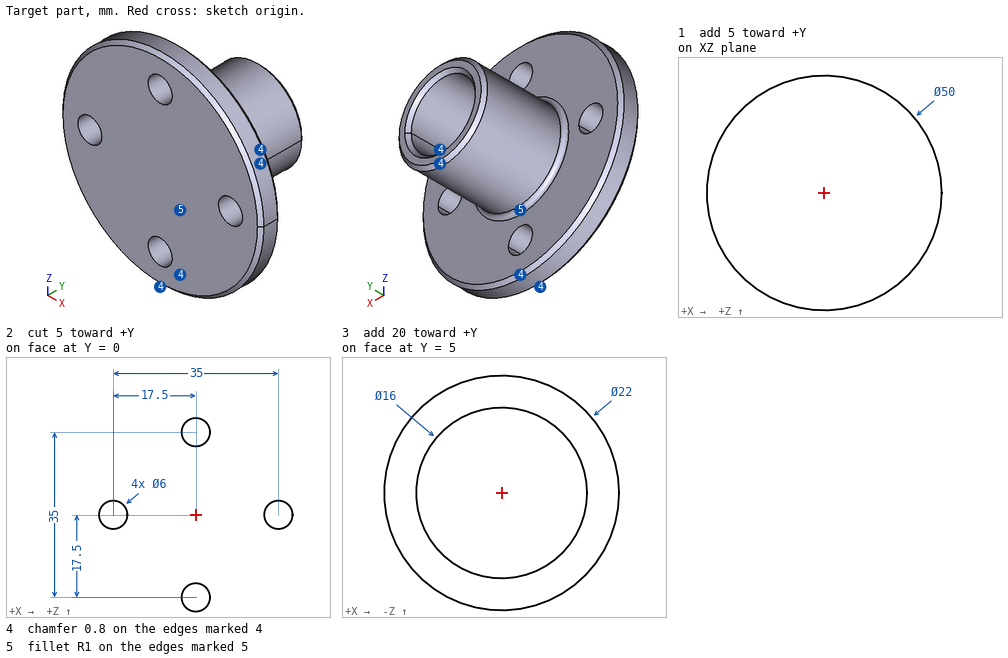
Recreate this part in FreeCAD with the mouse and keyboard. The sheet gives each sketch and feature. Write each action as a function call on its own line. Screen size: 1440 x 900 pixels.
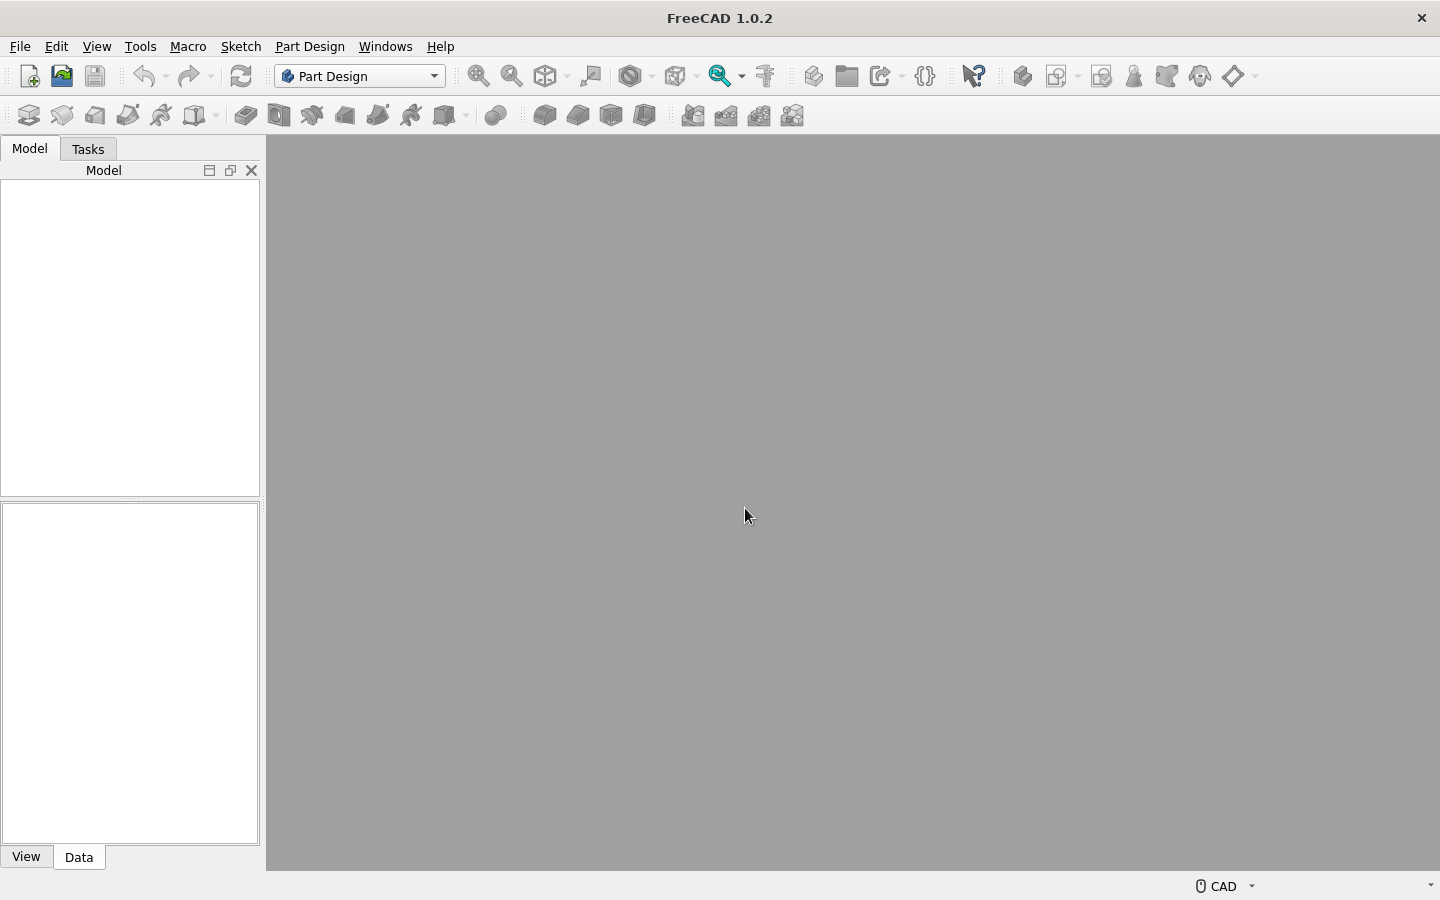
click(29, 76)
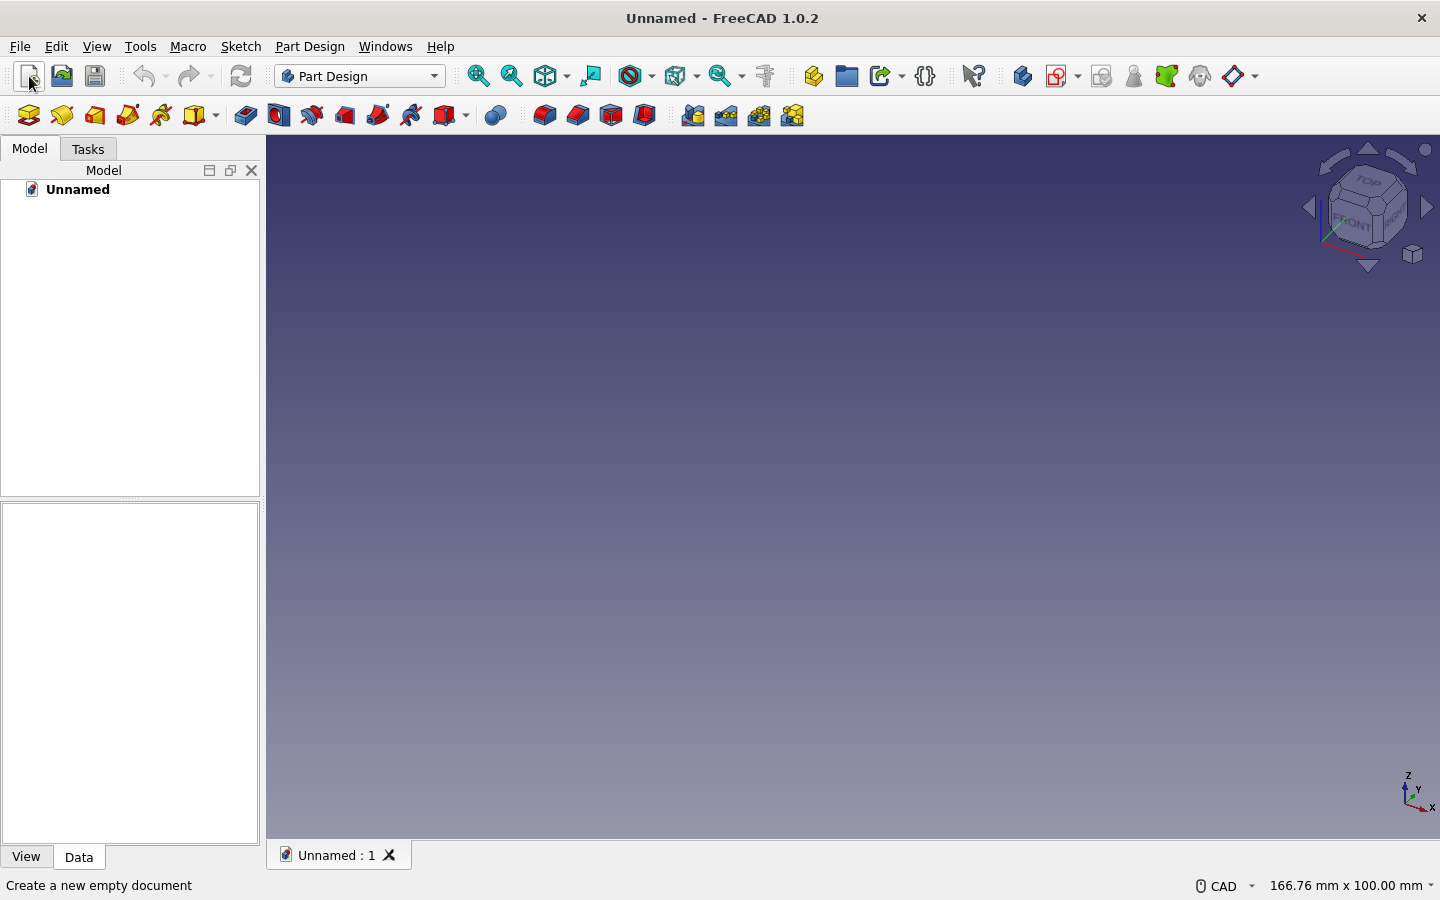
click(1056, 76)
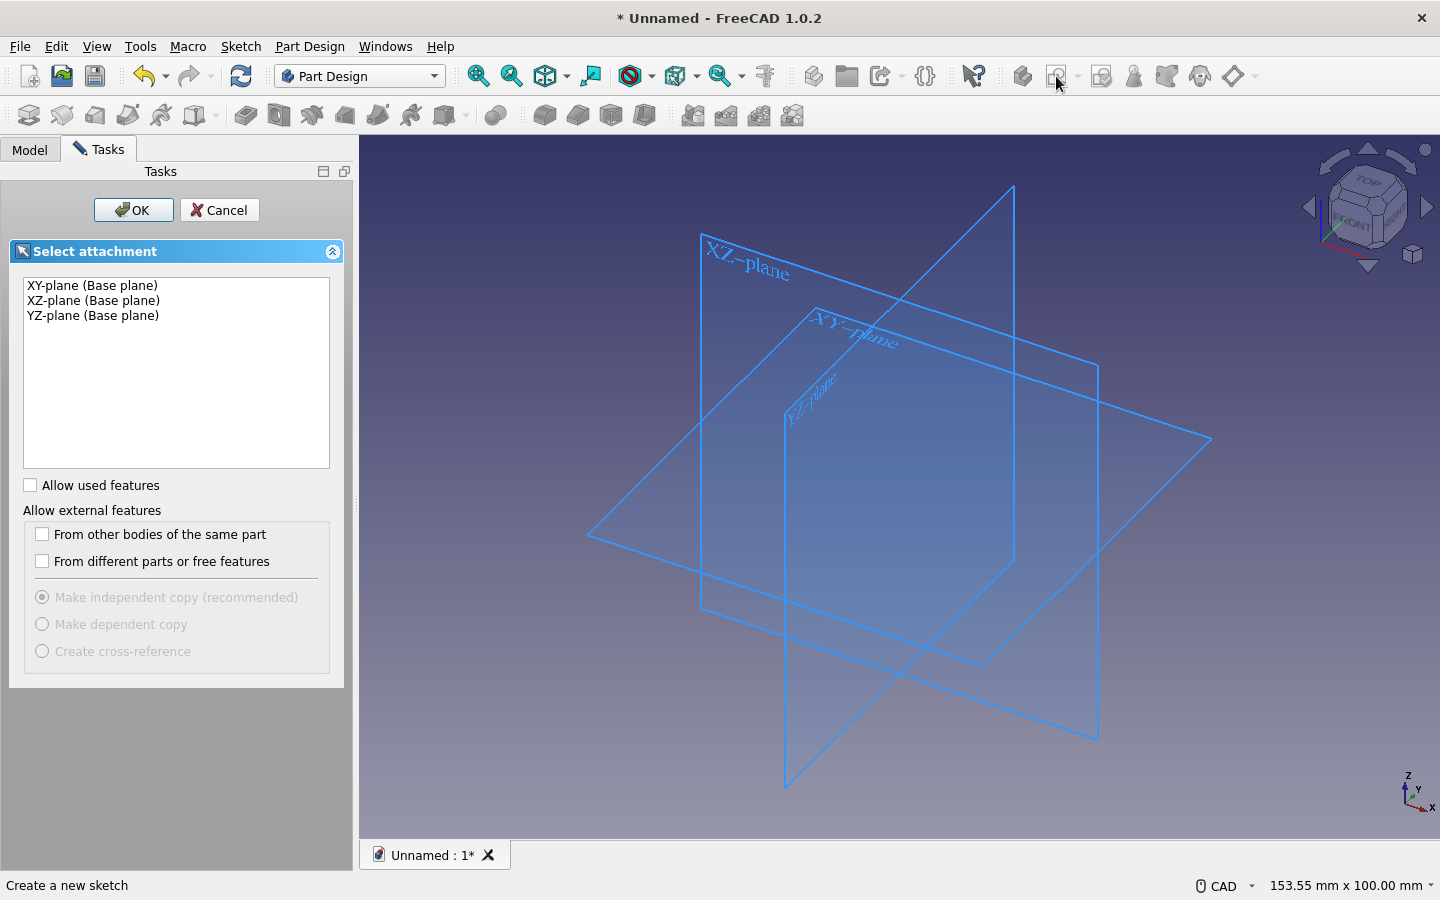
click(84, 300)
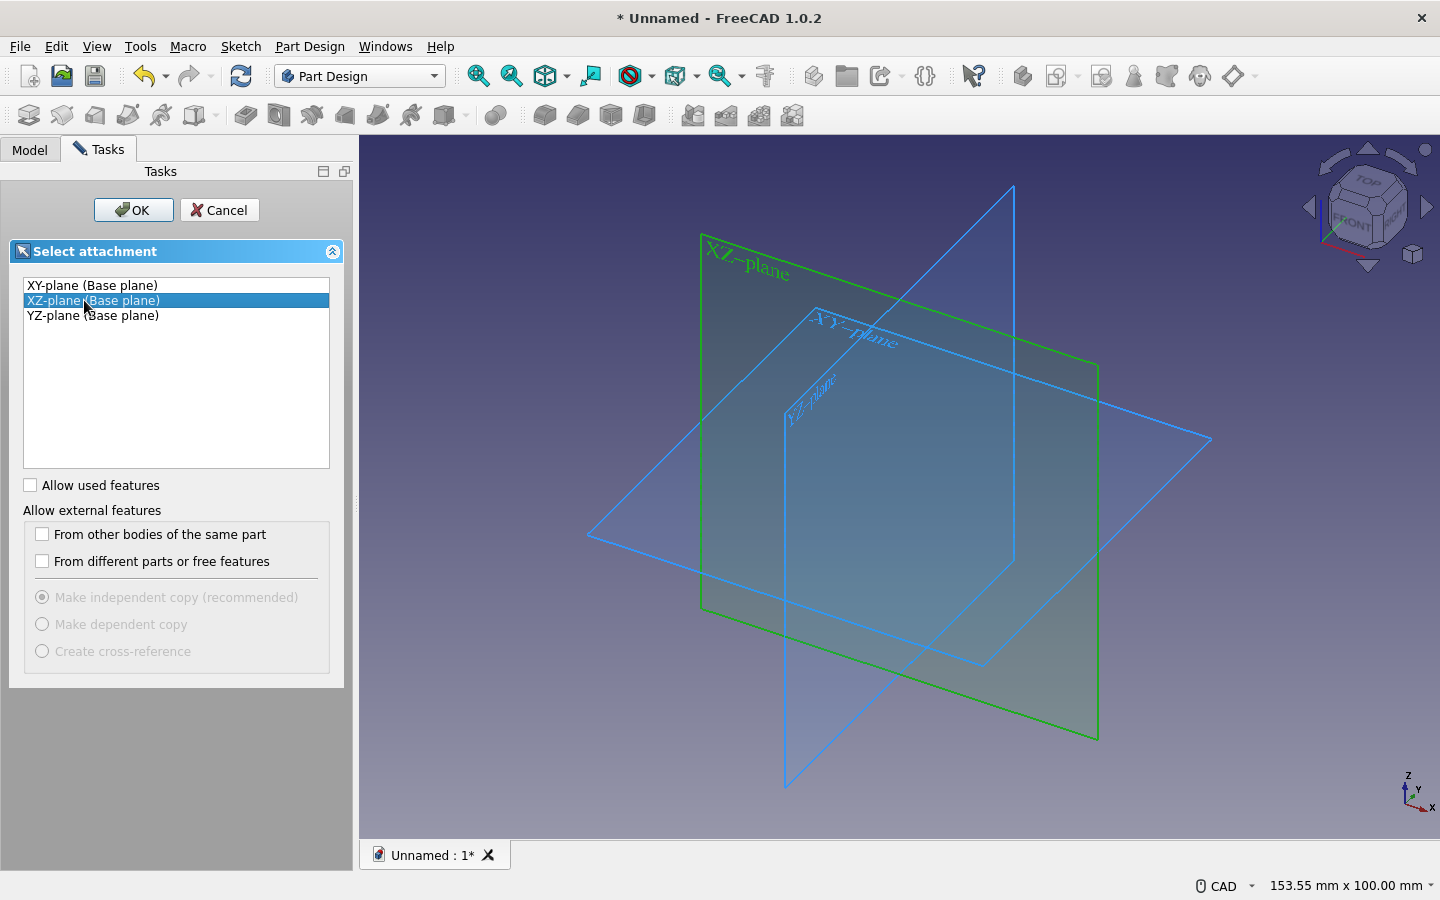
click(134, 210)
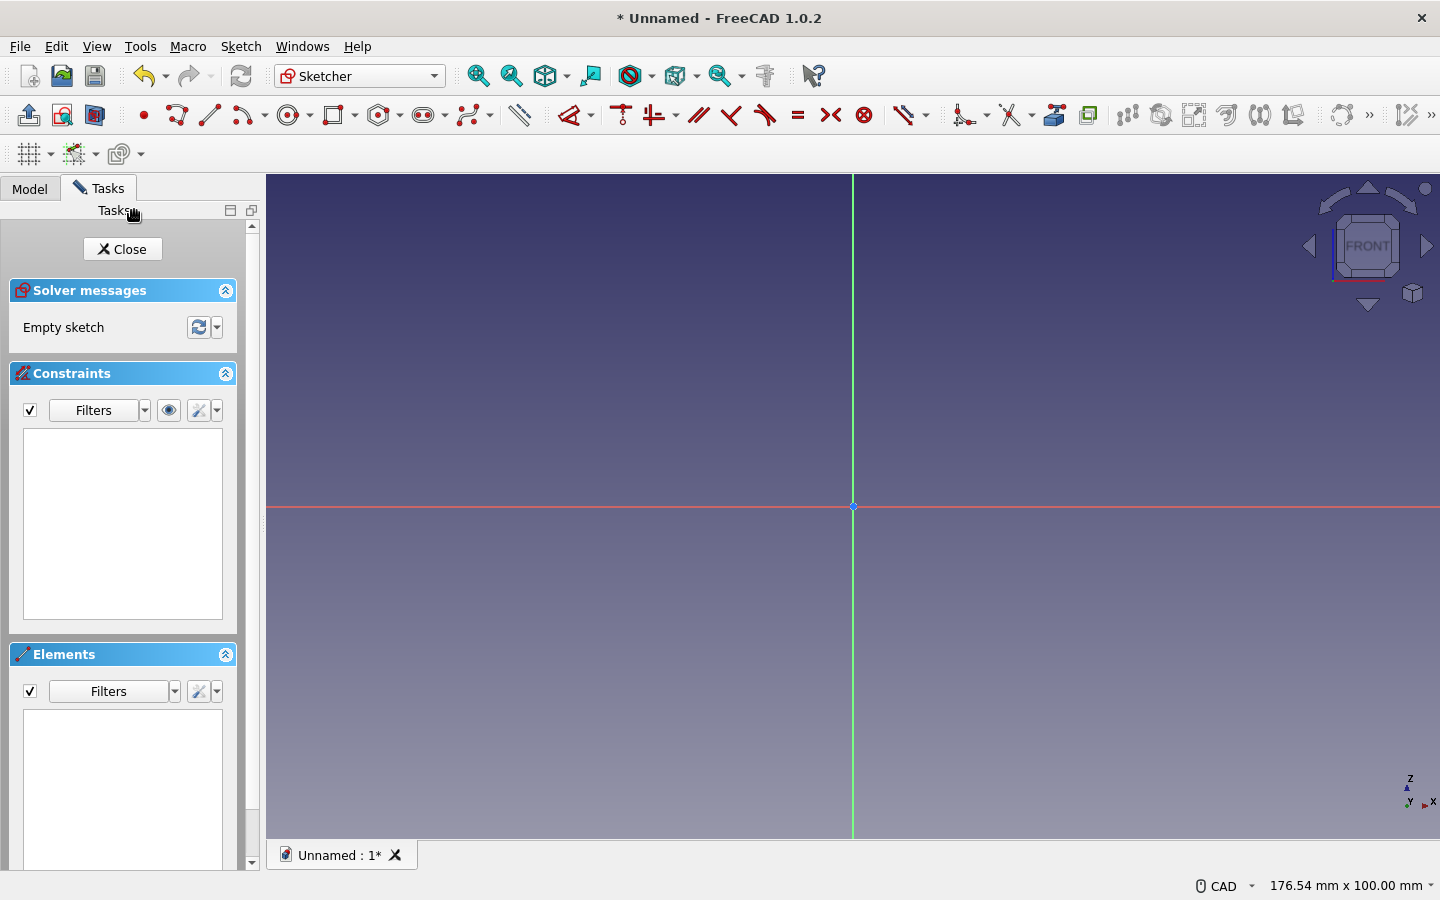
click(288, 116)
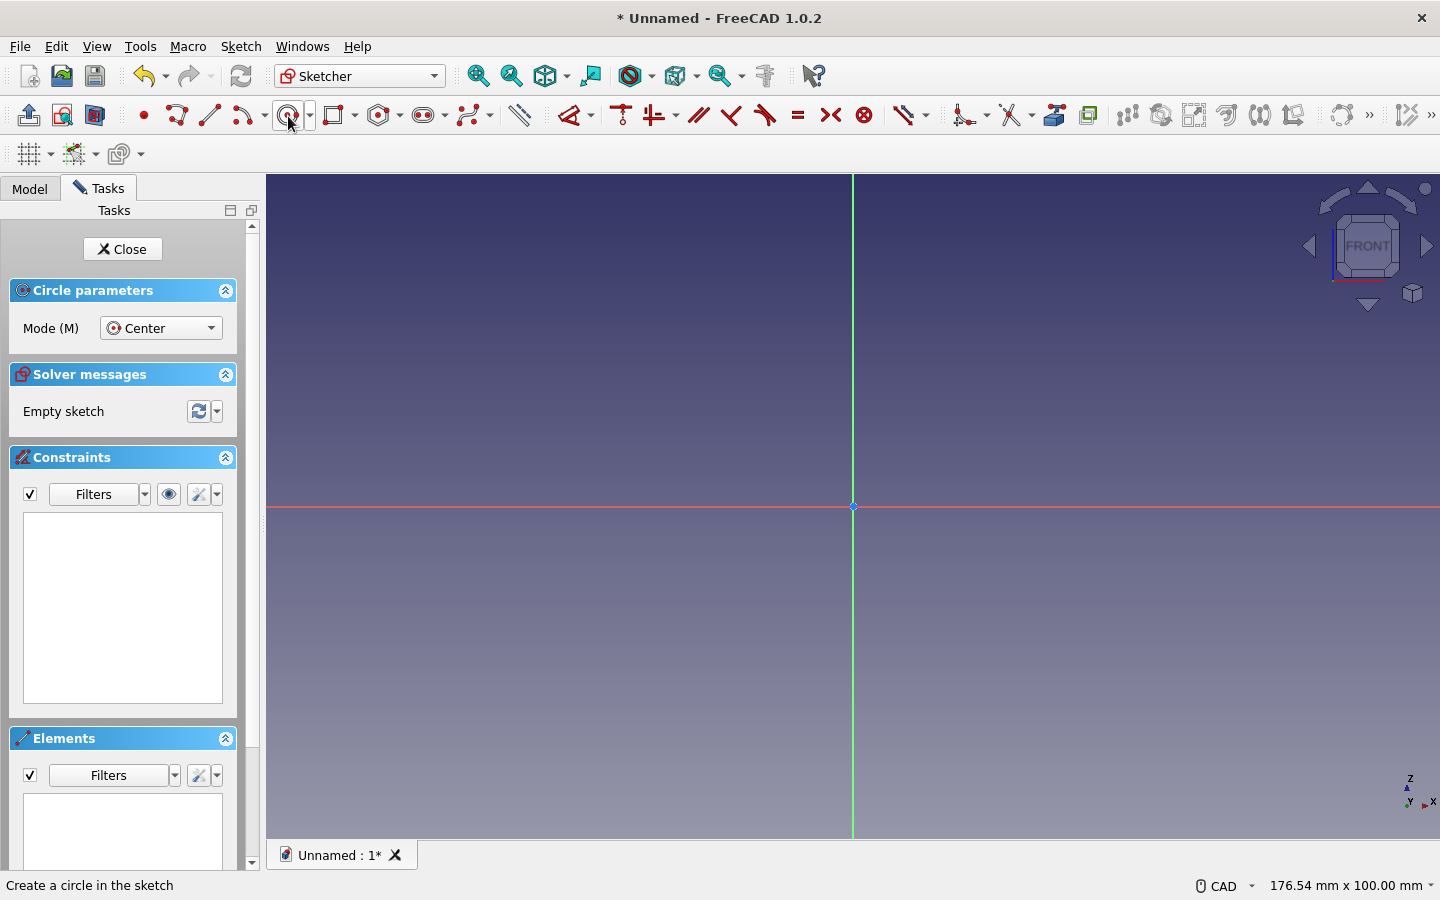
click(853, 506)
click(971, 389)
key(Escape)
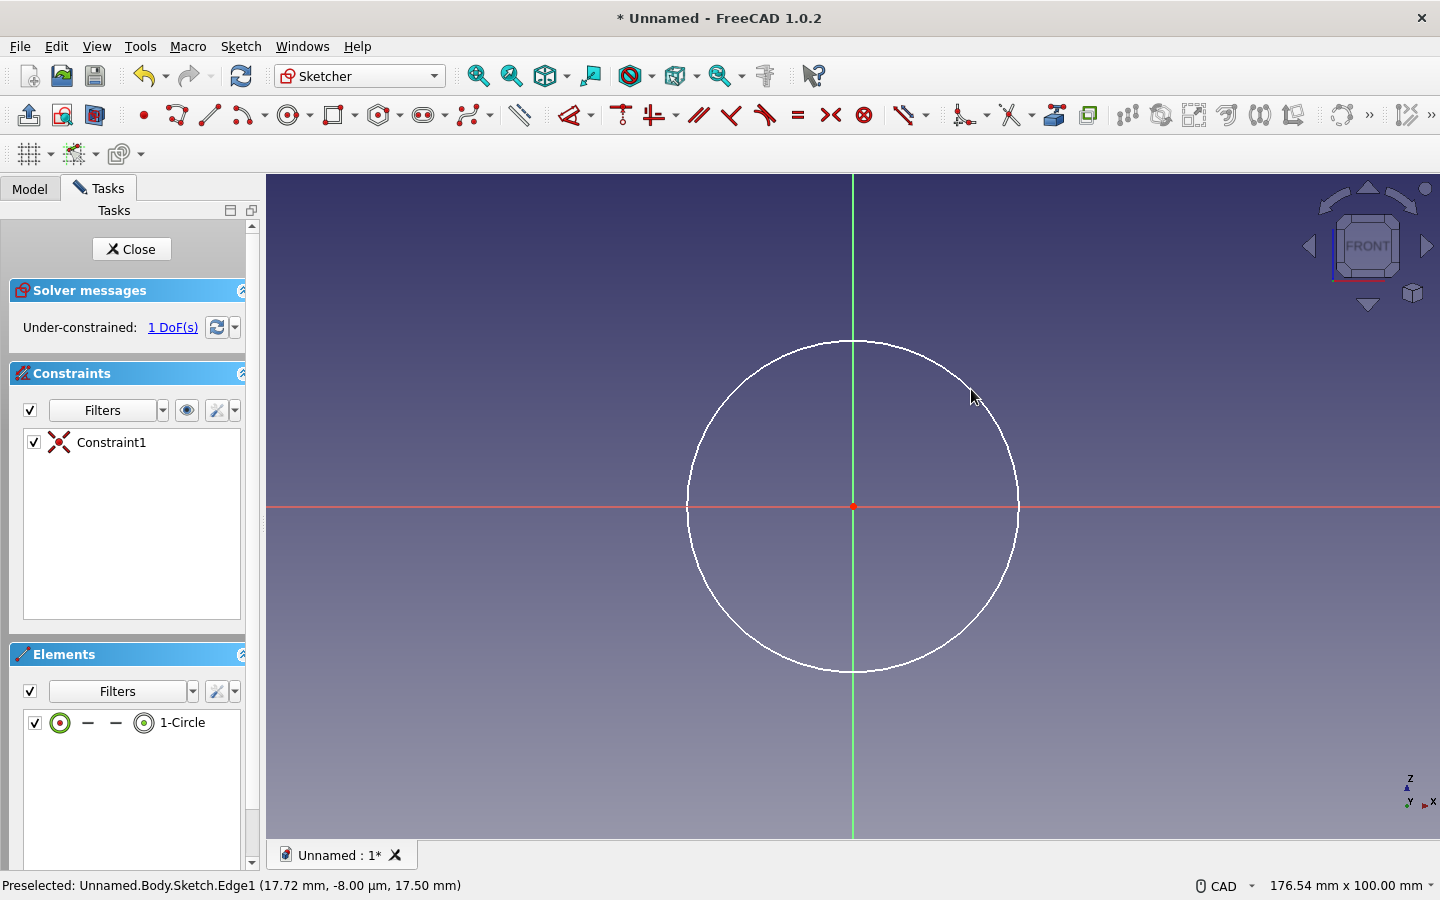
click(568, 116)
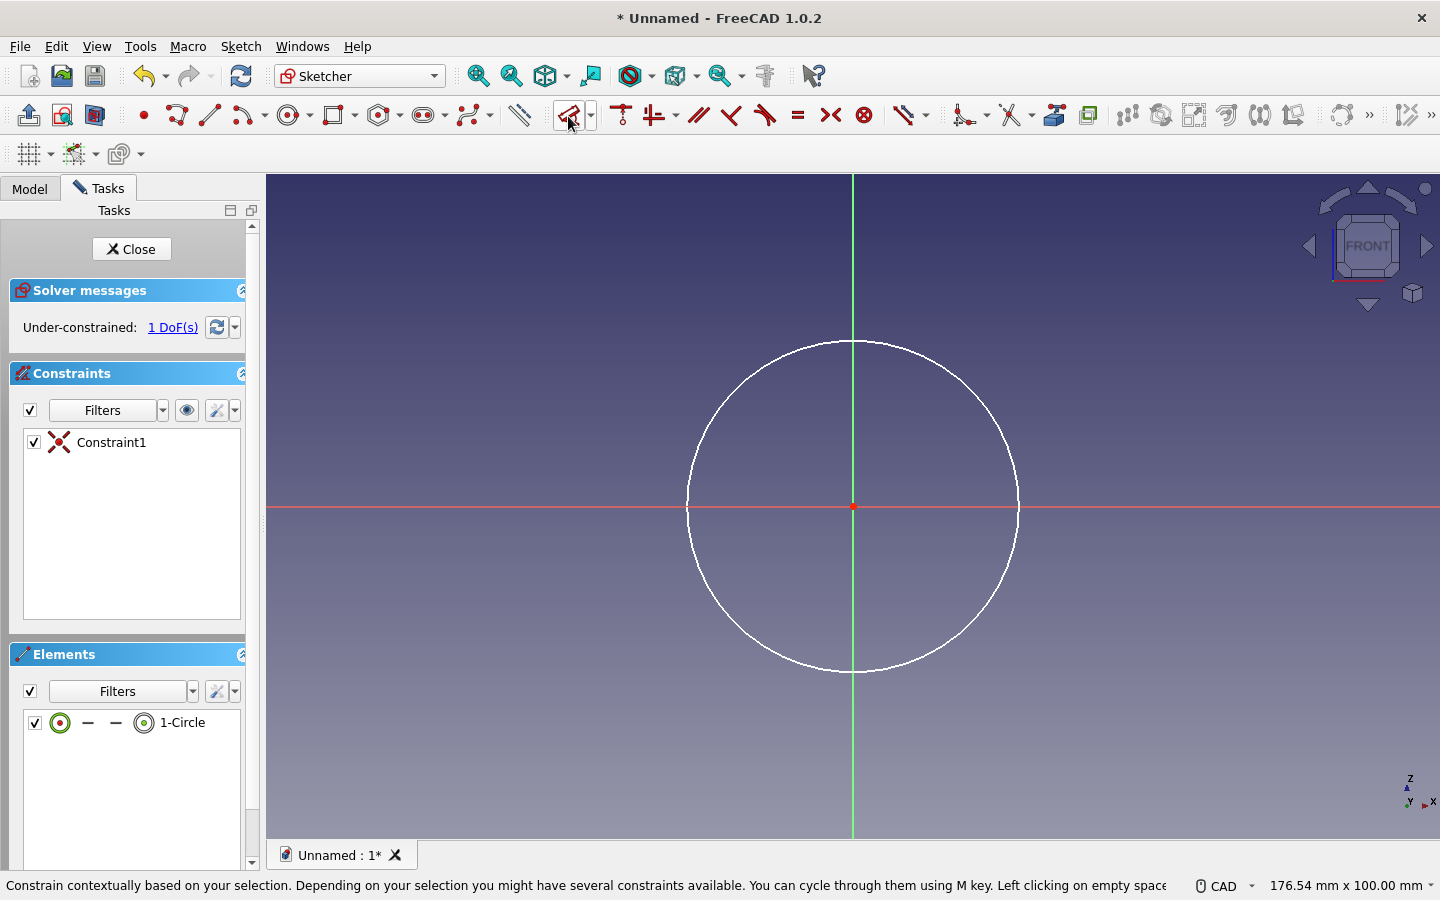
click(970, 389)
click(993, 366)